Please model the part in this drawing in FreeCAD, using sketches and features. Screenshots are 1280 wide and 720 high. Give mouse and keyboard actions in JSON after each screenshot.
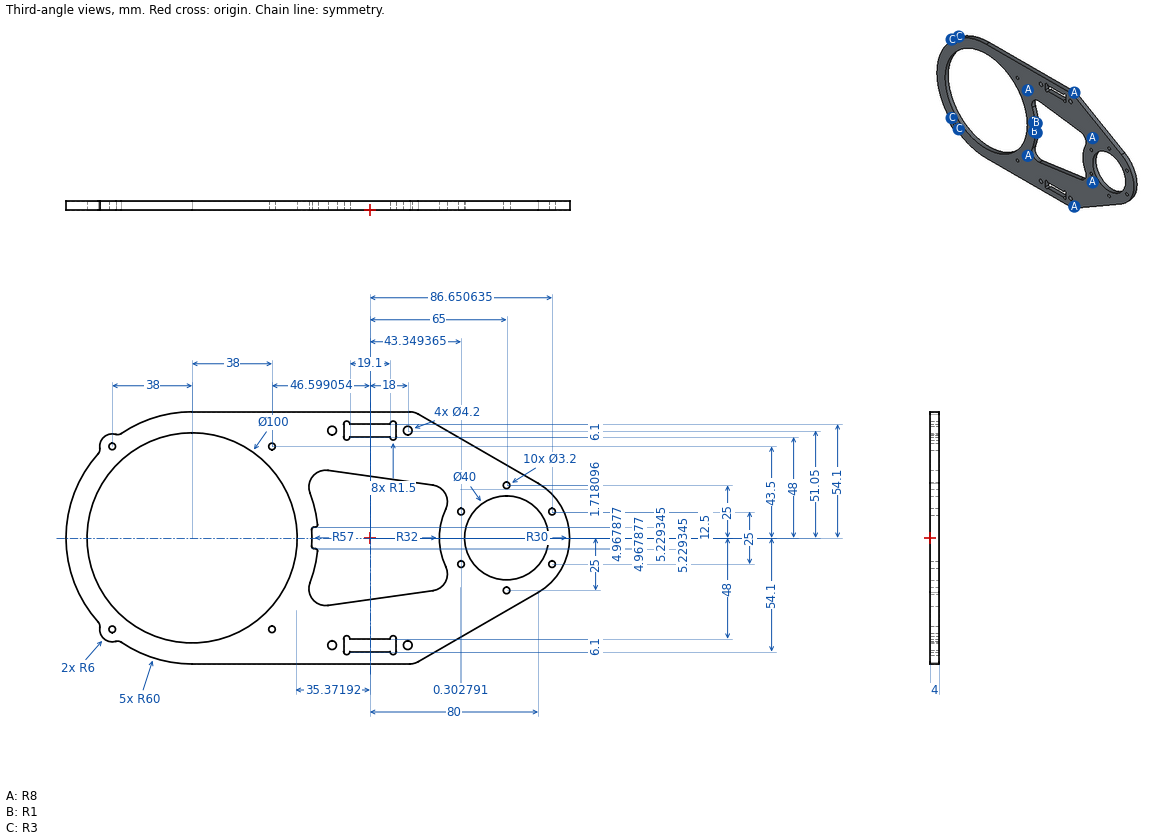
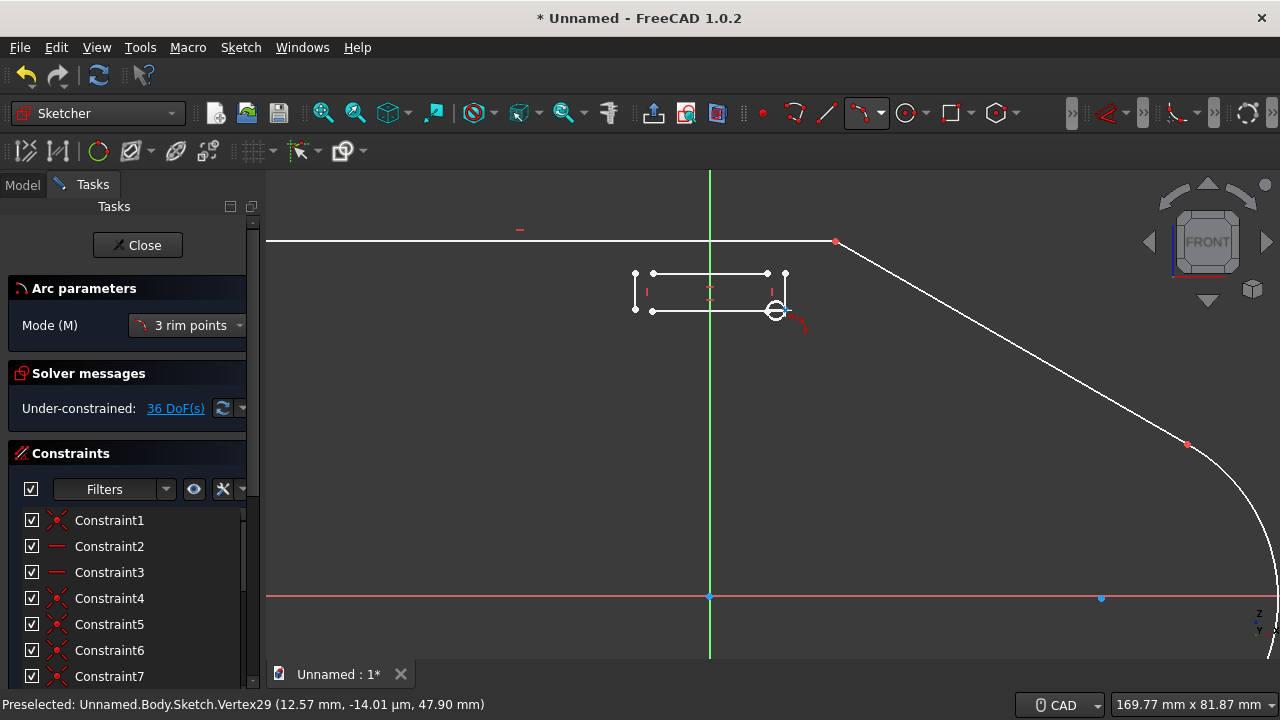
{"action": "scroll", "coordinate": [776, 318], "scroll_direction": "up", "scroll_amount": 3}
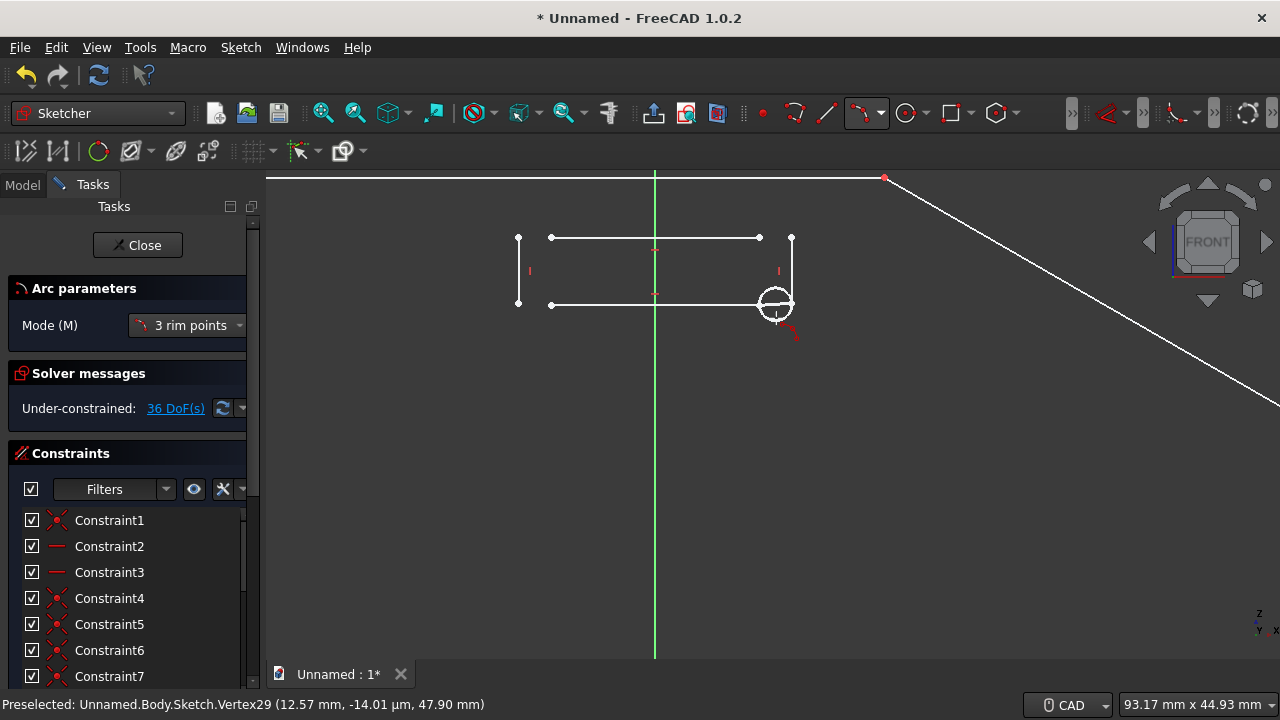
{"action": "left_click", "coordinate": [775, 318]}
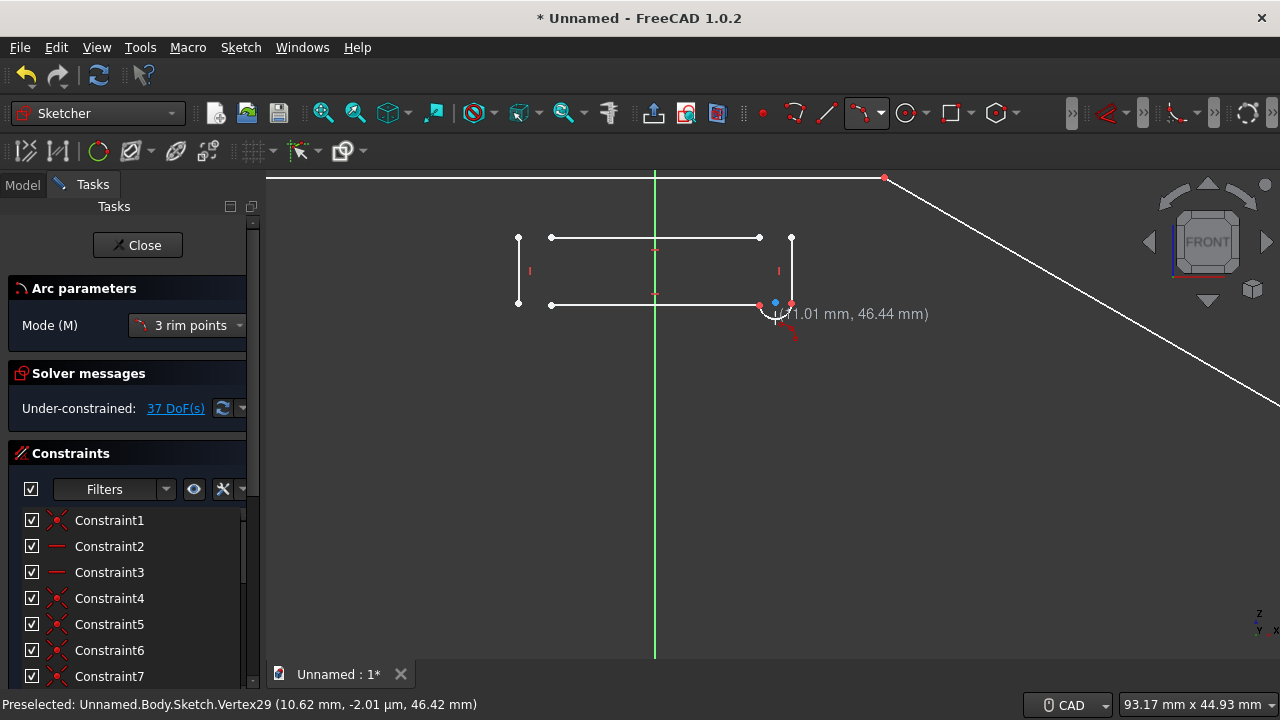
{"action": "left_click", "coordinate": [792, 238]}
{"action": "left_click", "coordinate": [759, 238]}
{"action": "left_click", "coordinate": [775, 219]}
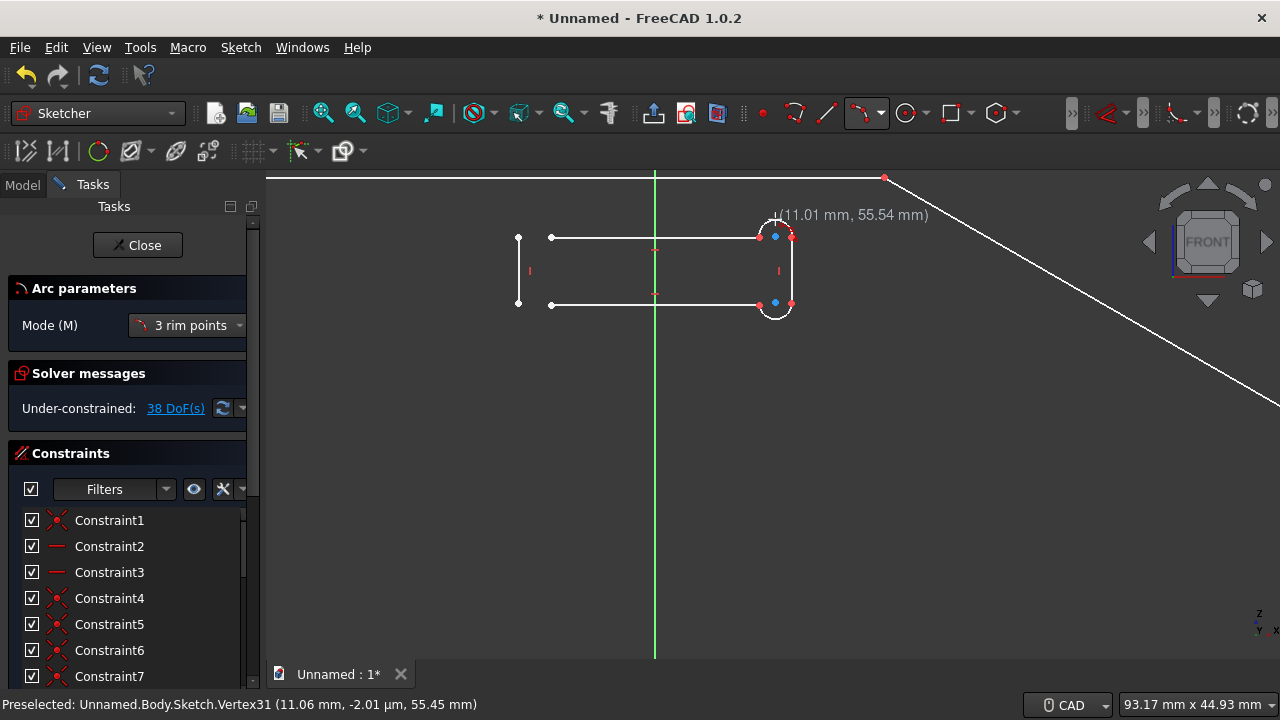
{"action": "left_click", "coordinate": [551, 238]}
{"action": "left_click", "coordinate": [519, 238]}
{"action": "left_click", "coordinate": [535, 219]}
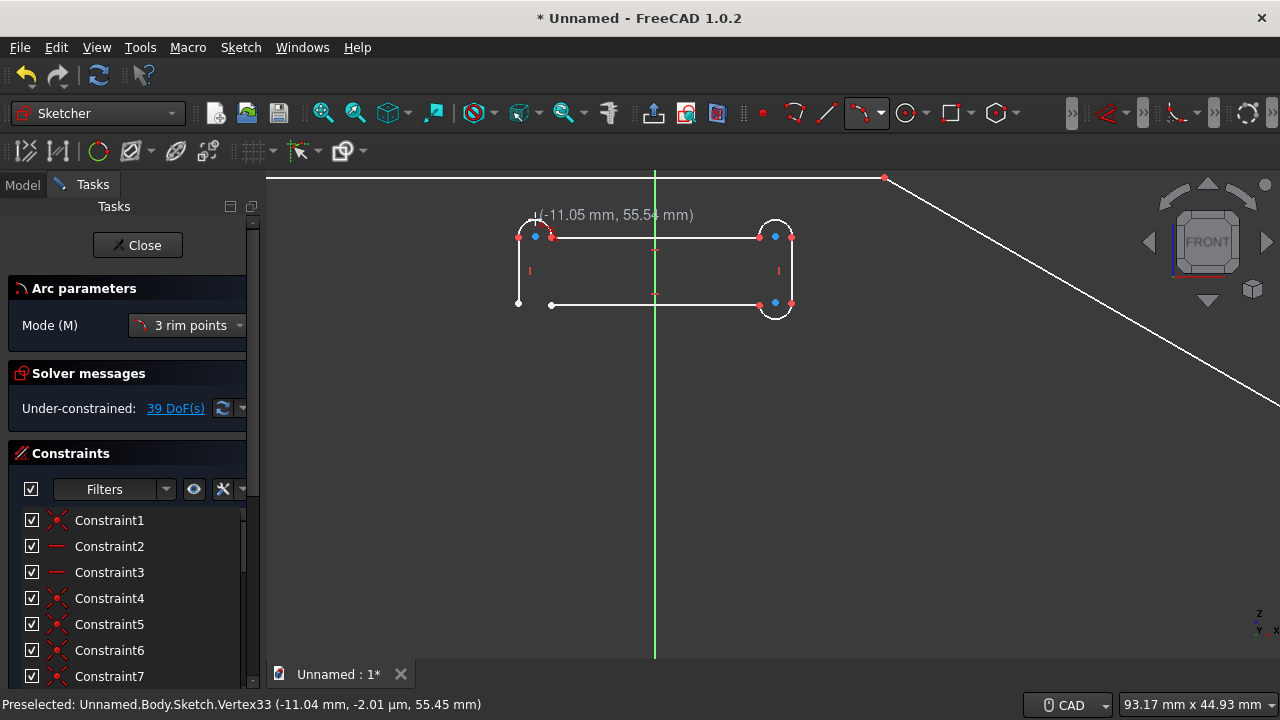
{"action": "left_click", "coordinate": [519, 303]}
{"action": "left_click", "coordinate": [551, 305]}
{"action": "left_click", "coordinate": [535, 318]}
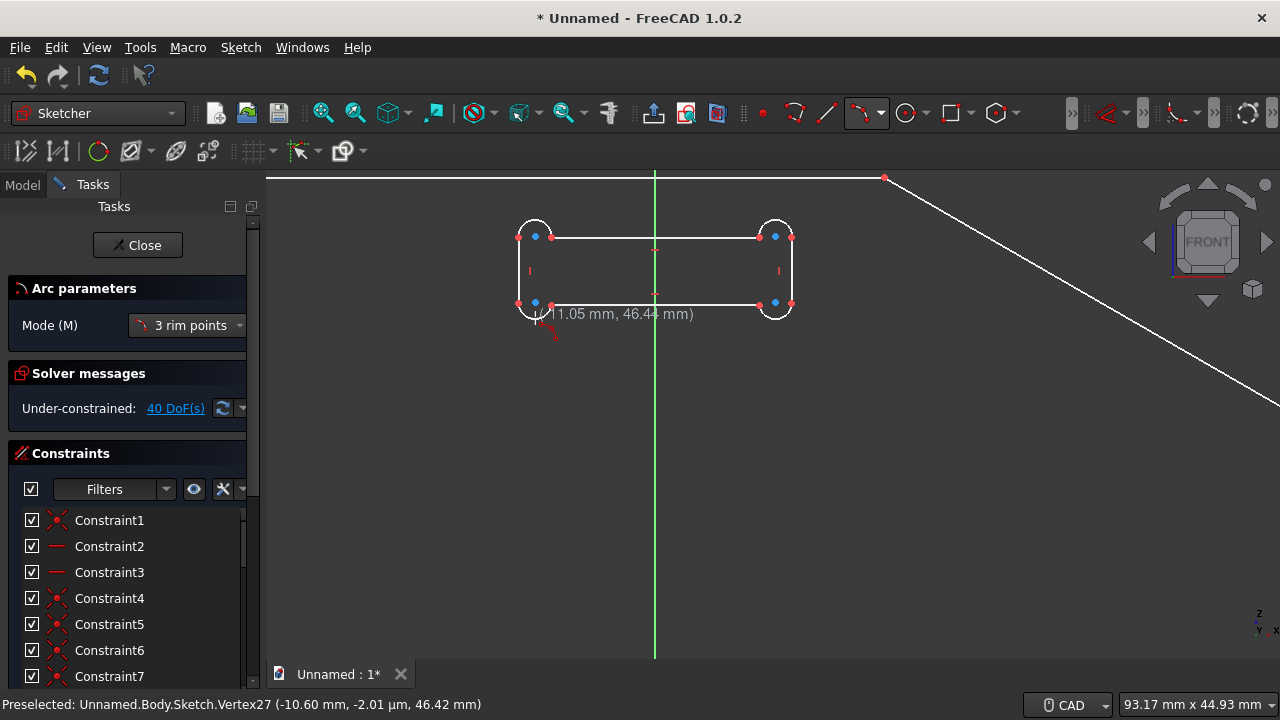
{"action": "left_click", "coordinate": [828, 114]}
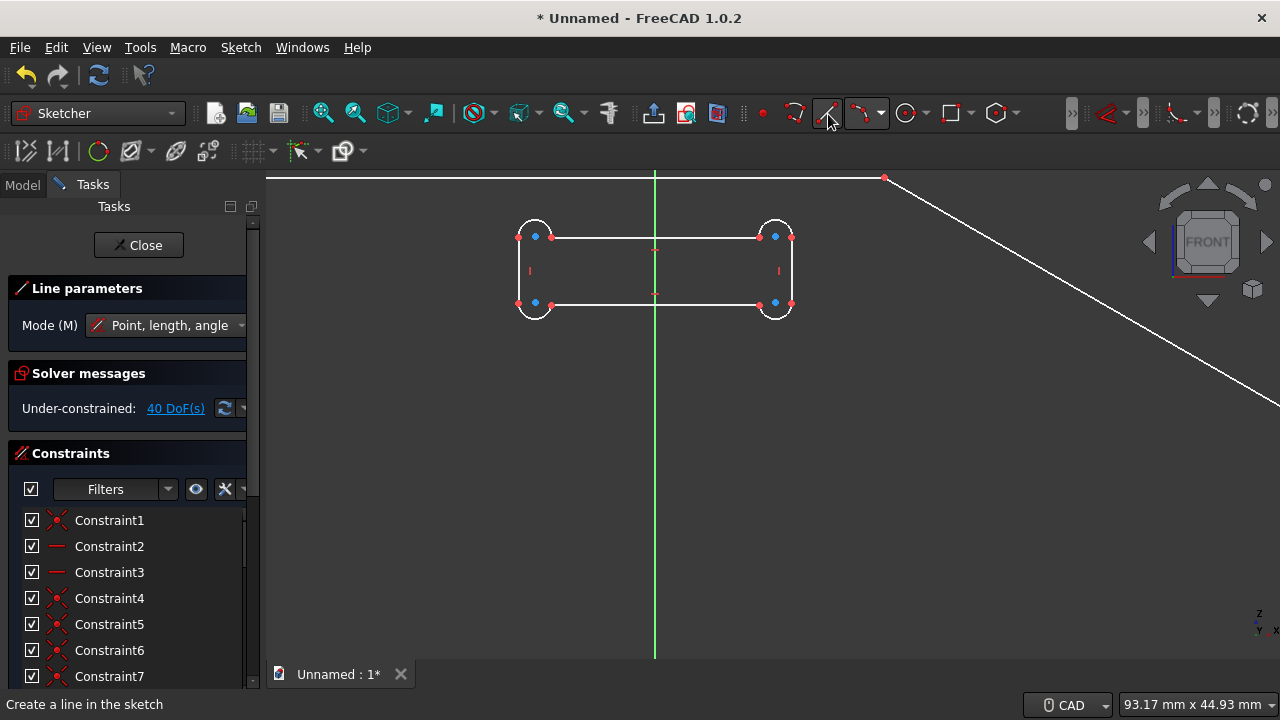
{"action": "scroll", "coordinate": [785, 311], "scroll_direction": "down", "scroll_amount": 8}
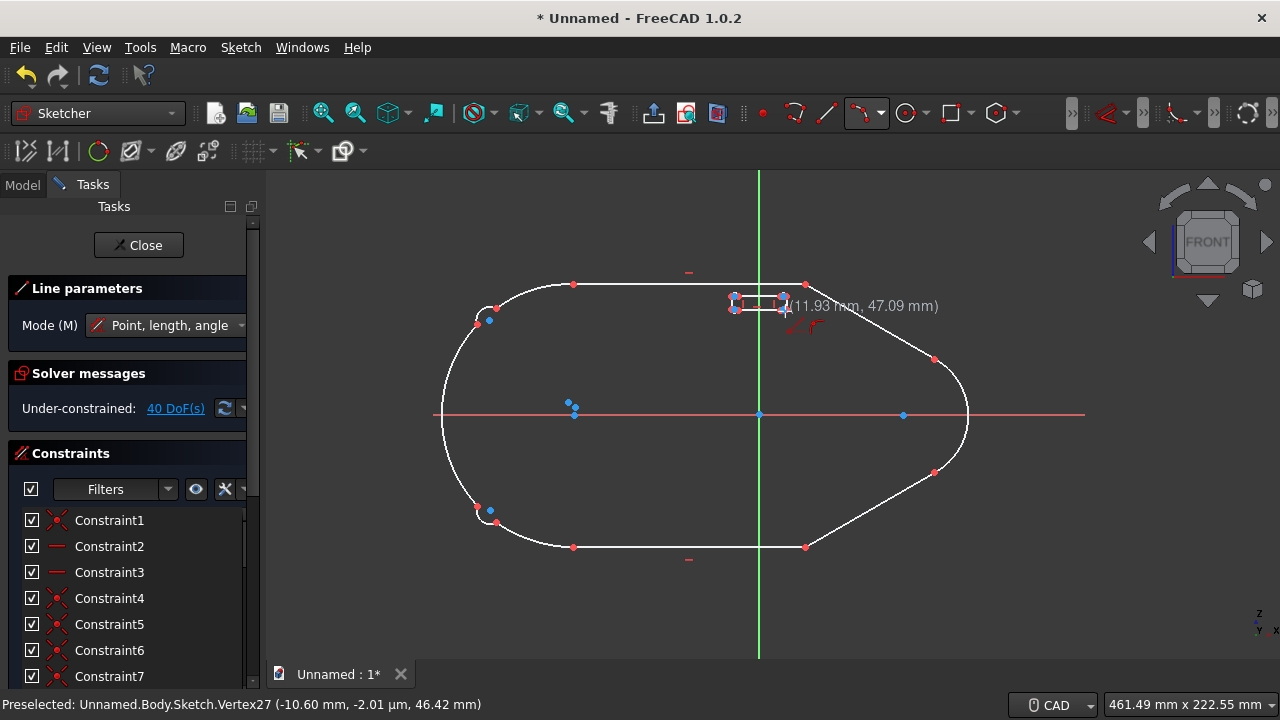
{"action": "left_click", "coordinate": [681, 490]}
{"action": "left_click", "coordinate": [854, 466]}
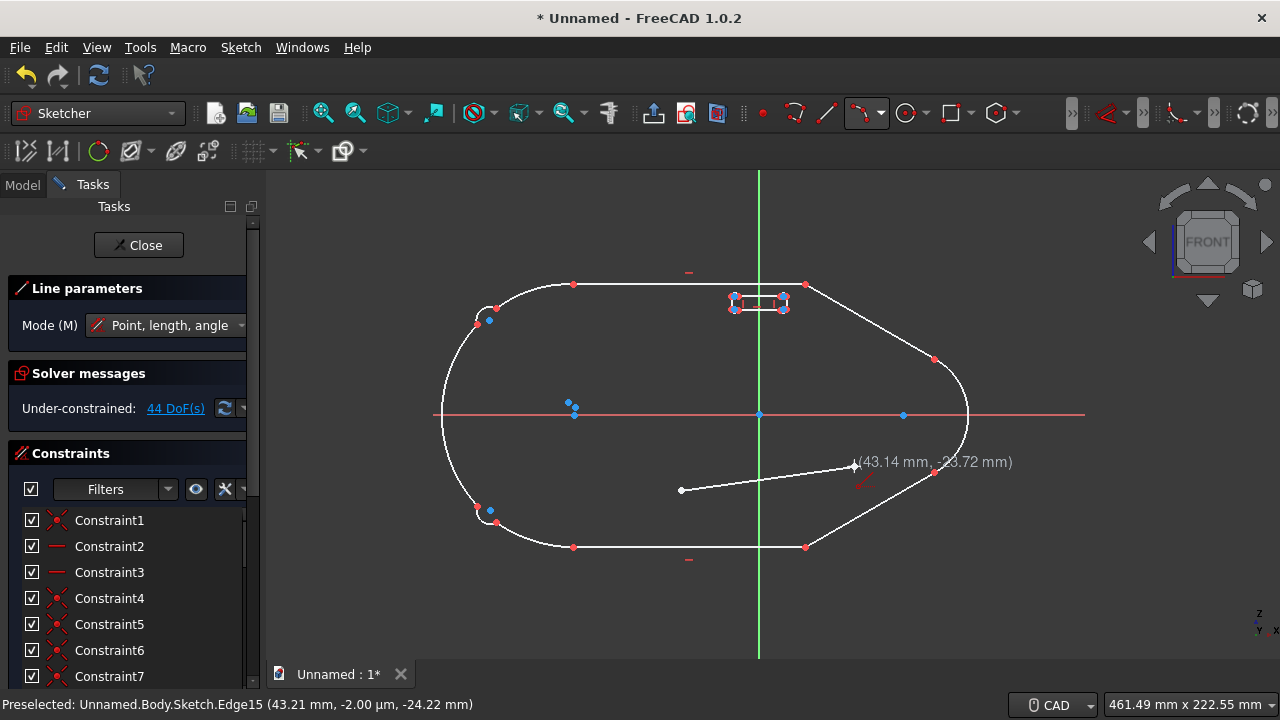
{"action": "left_click", "coordinate": [854, 364]}
{"action": "left_click", "coordinate": [681, 340]}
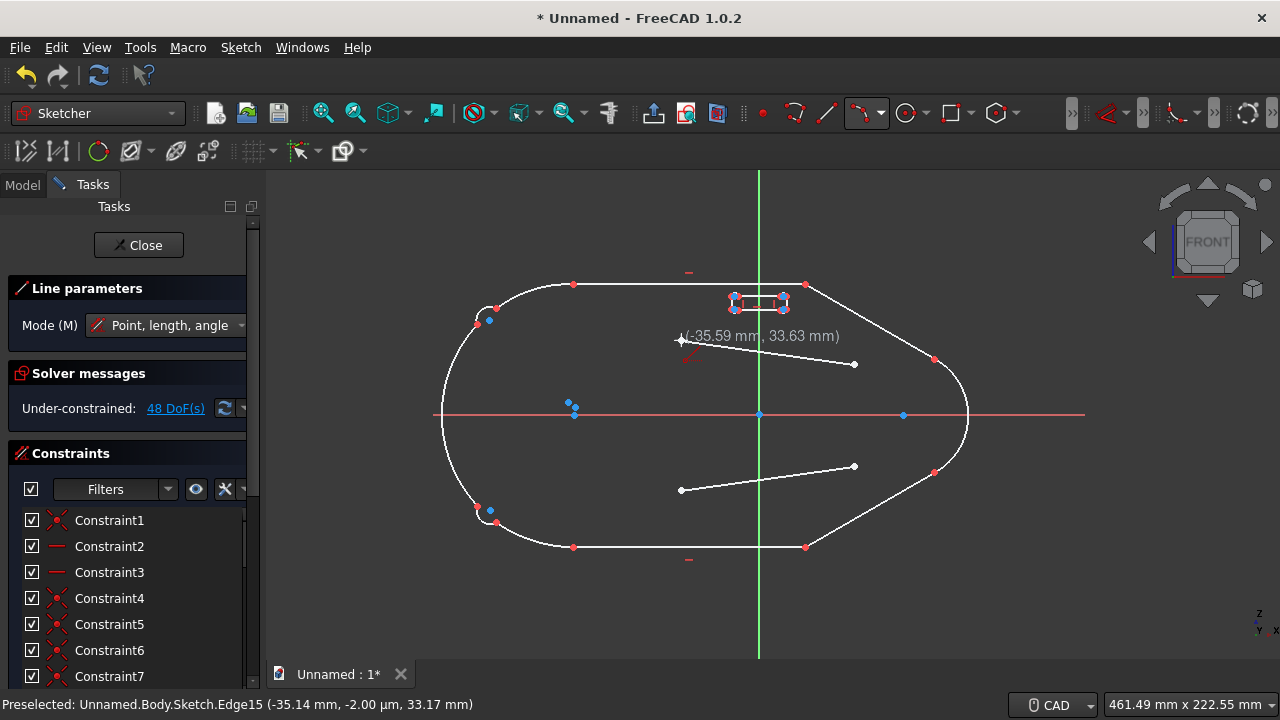
{"action": "scroll", "coordinate": [705, 403], "scroll_direction": "up", "scroll_amount": 2}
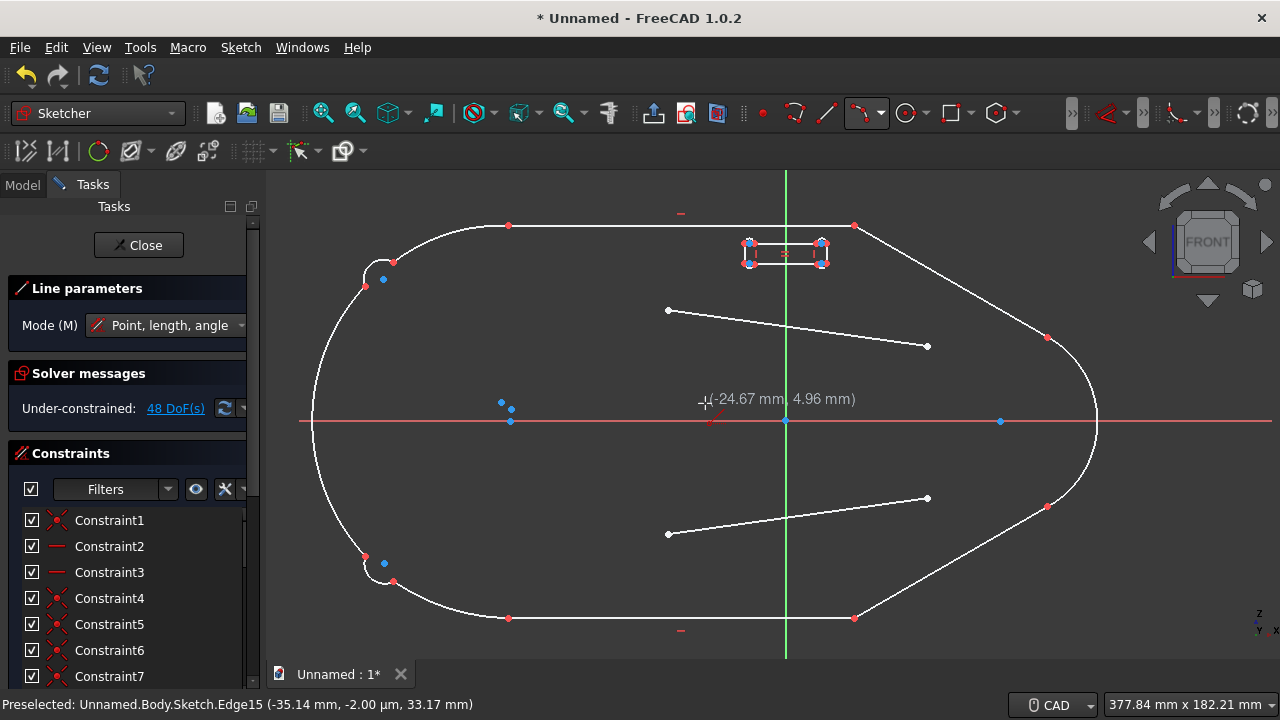
{"action": "left_click", "coordinate": [704, 403]}